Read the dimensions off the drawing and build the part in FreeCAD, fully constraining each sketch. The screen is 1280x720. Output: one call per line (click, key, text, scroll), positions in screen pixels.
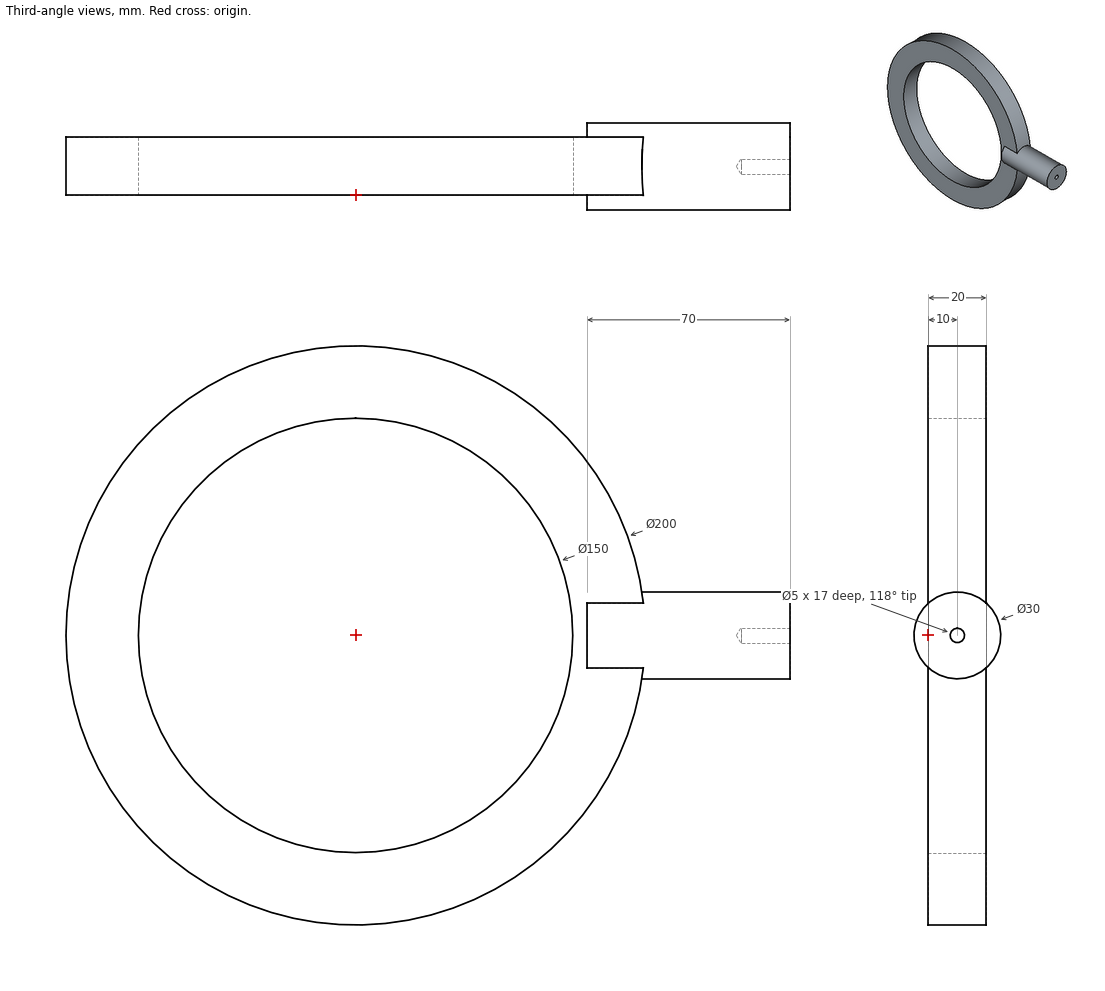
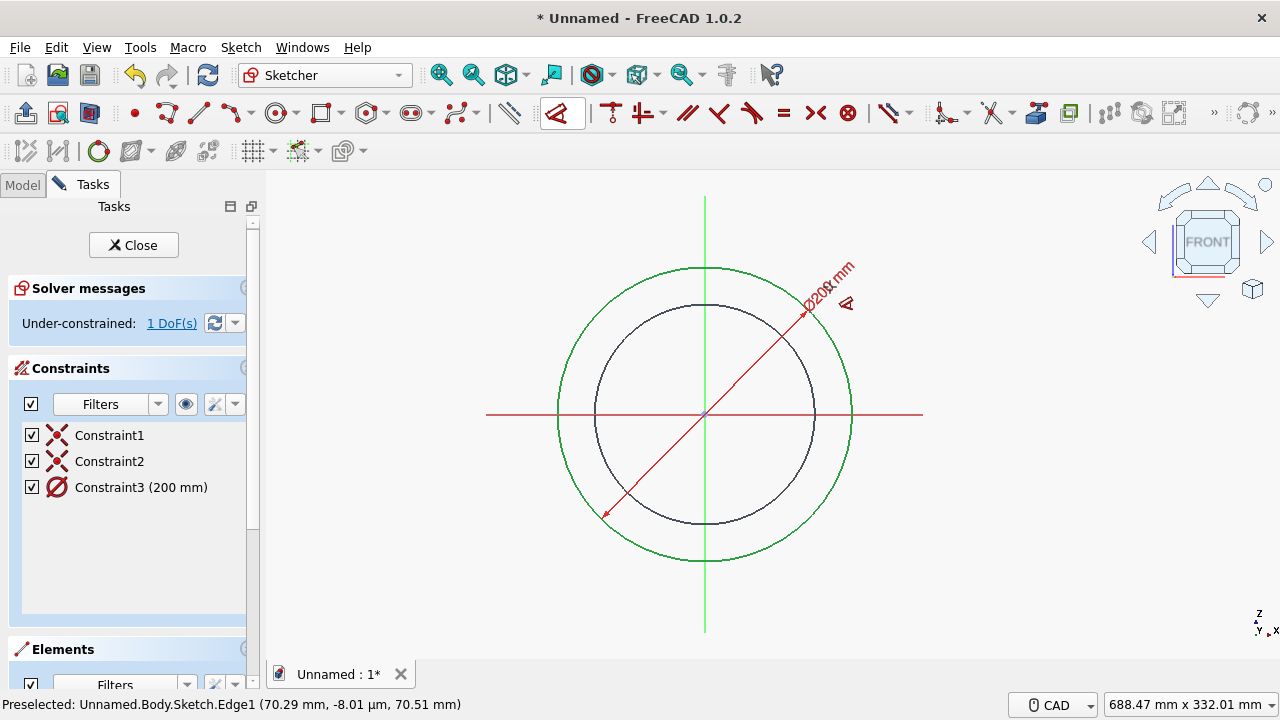
click(782, 336)
click(863, 367)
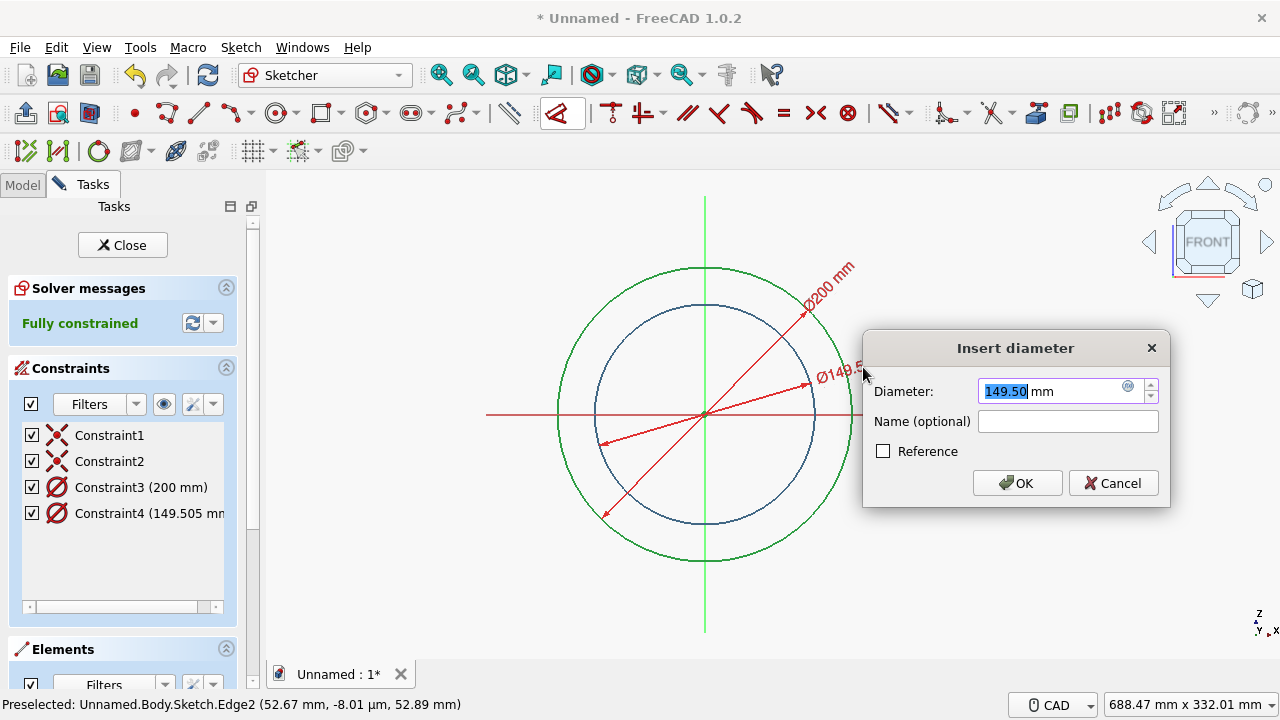
text(150)
key(Return)
key(Escape)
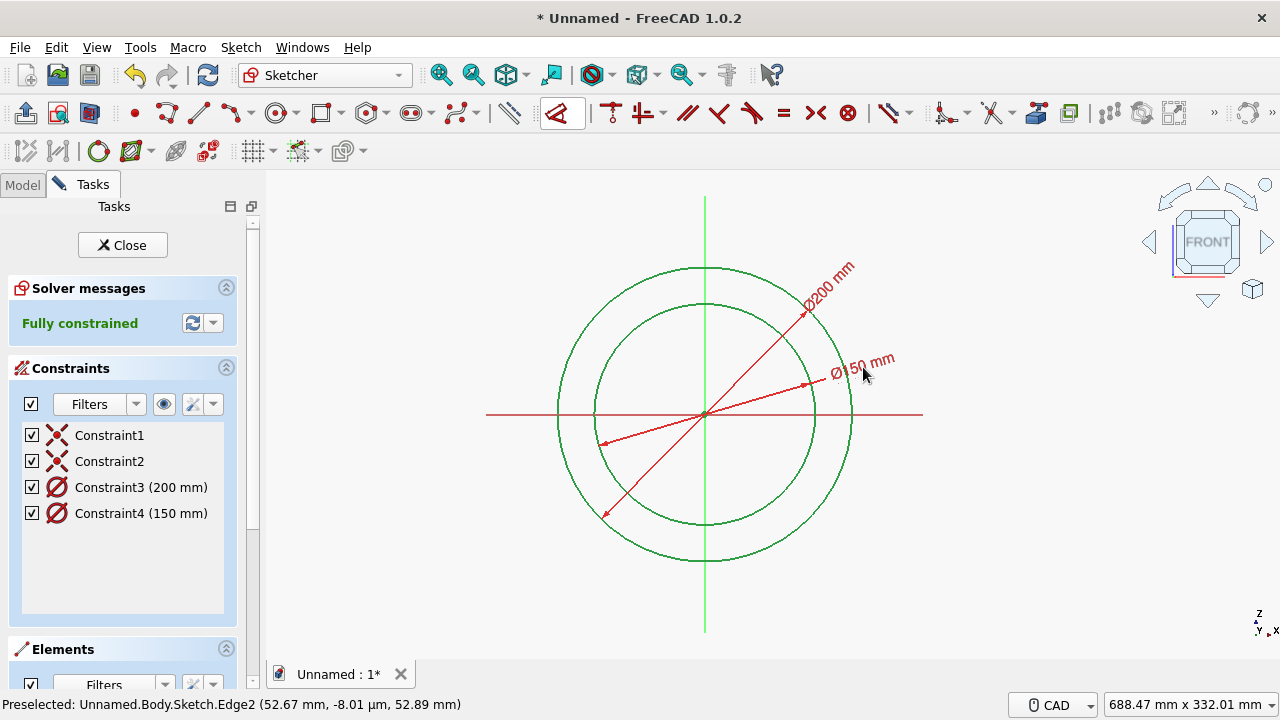
click(123, 245)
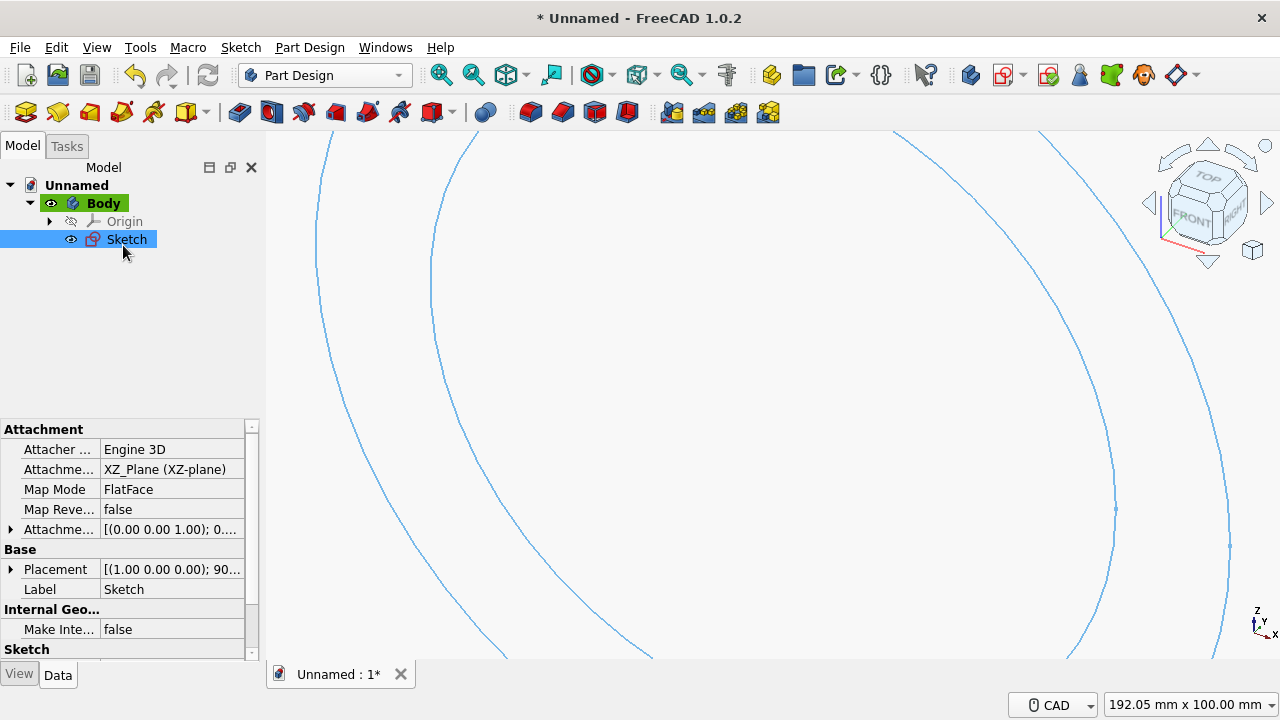
click(26, 112)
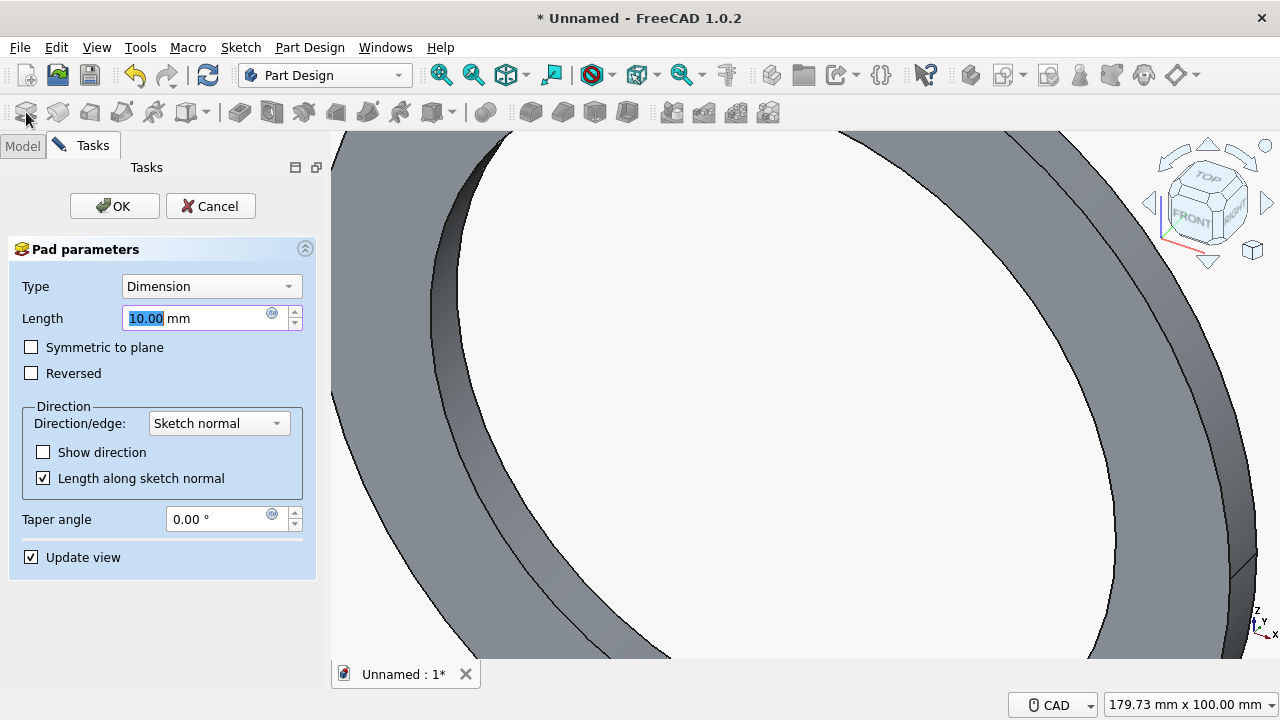
text(20)
key(Tab)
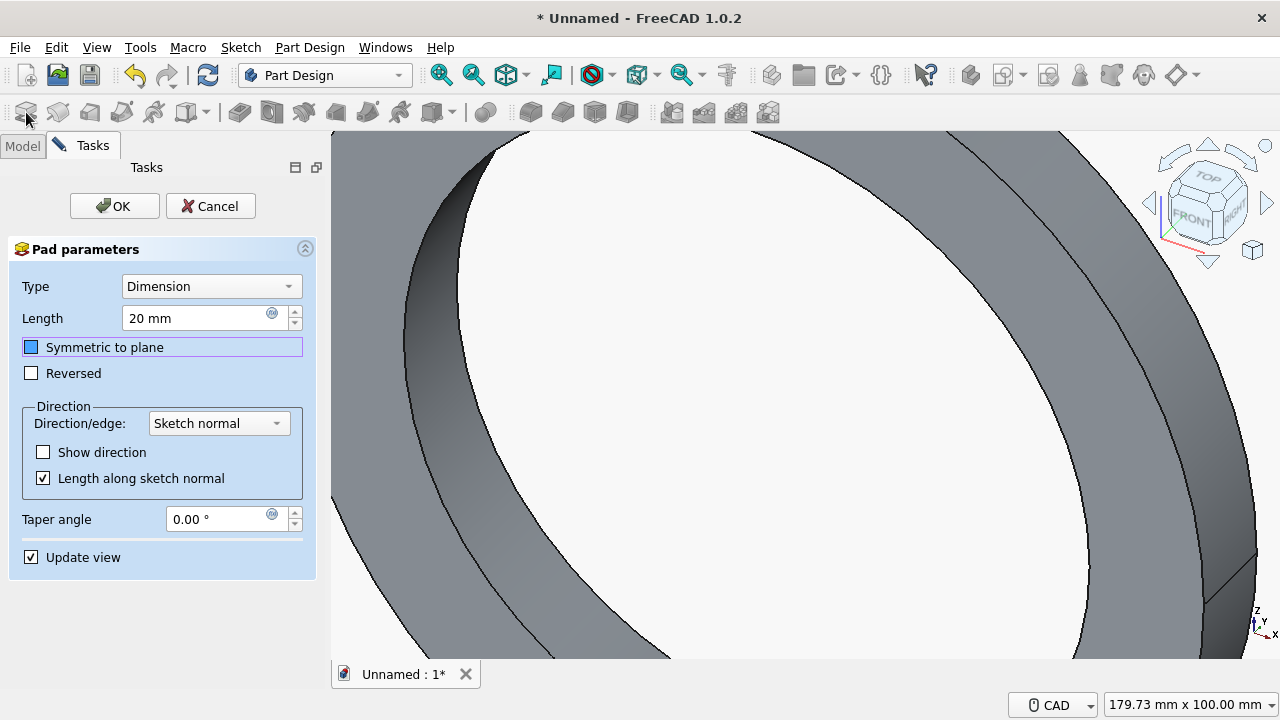
click(30, 373)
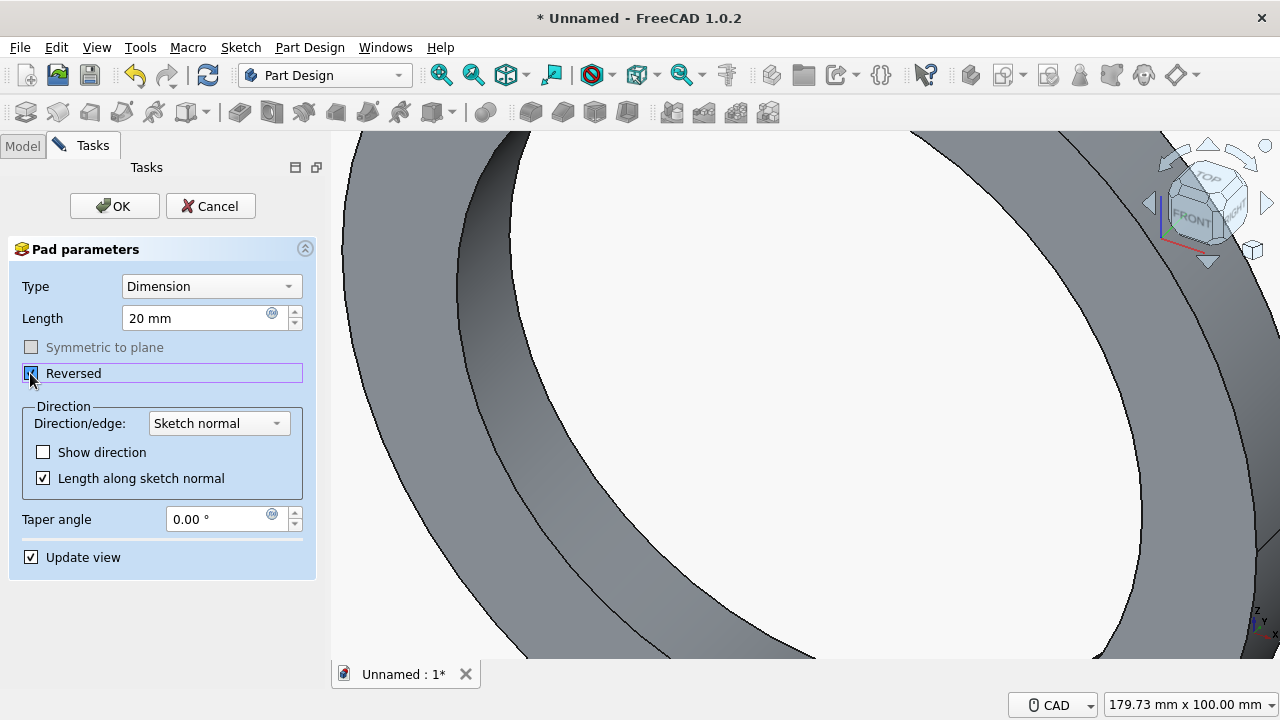
click(115, 206)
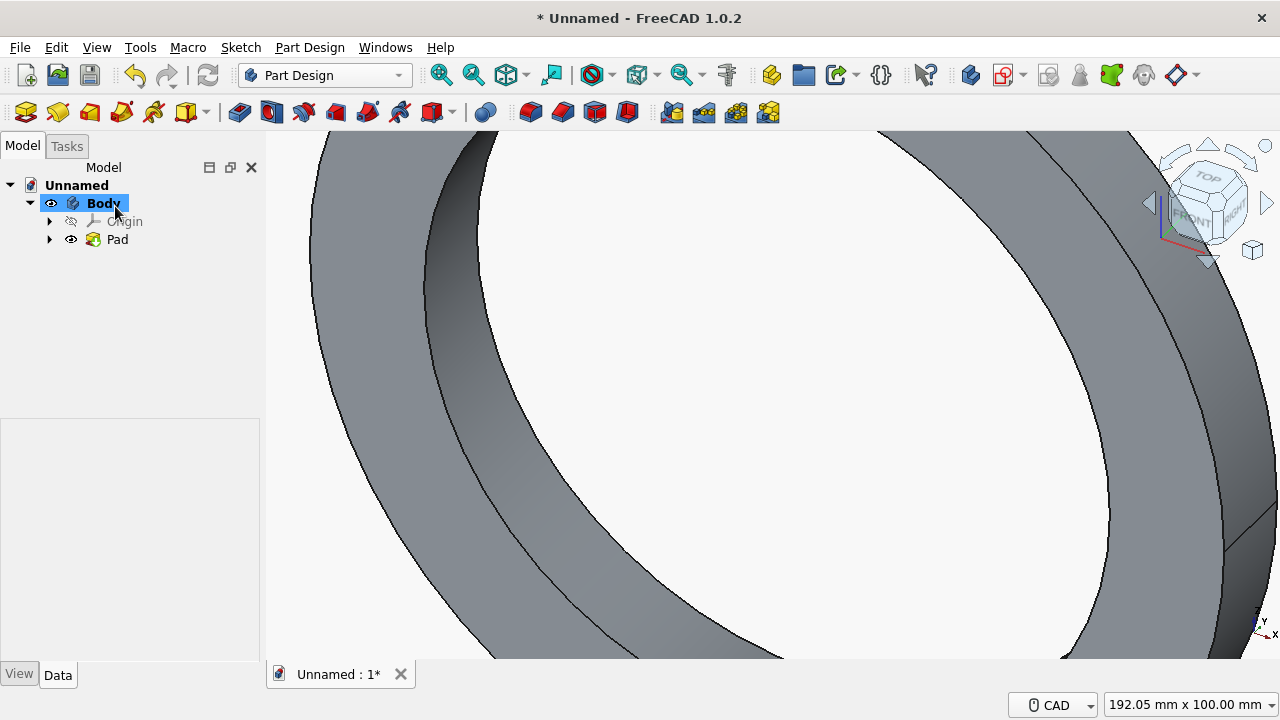
key(v)
key(f)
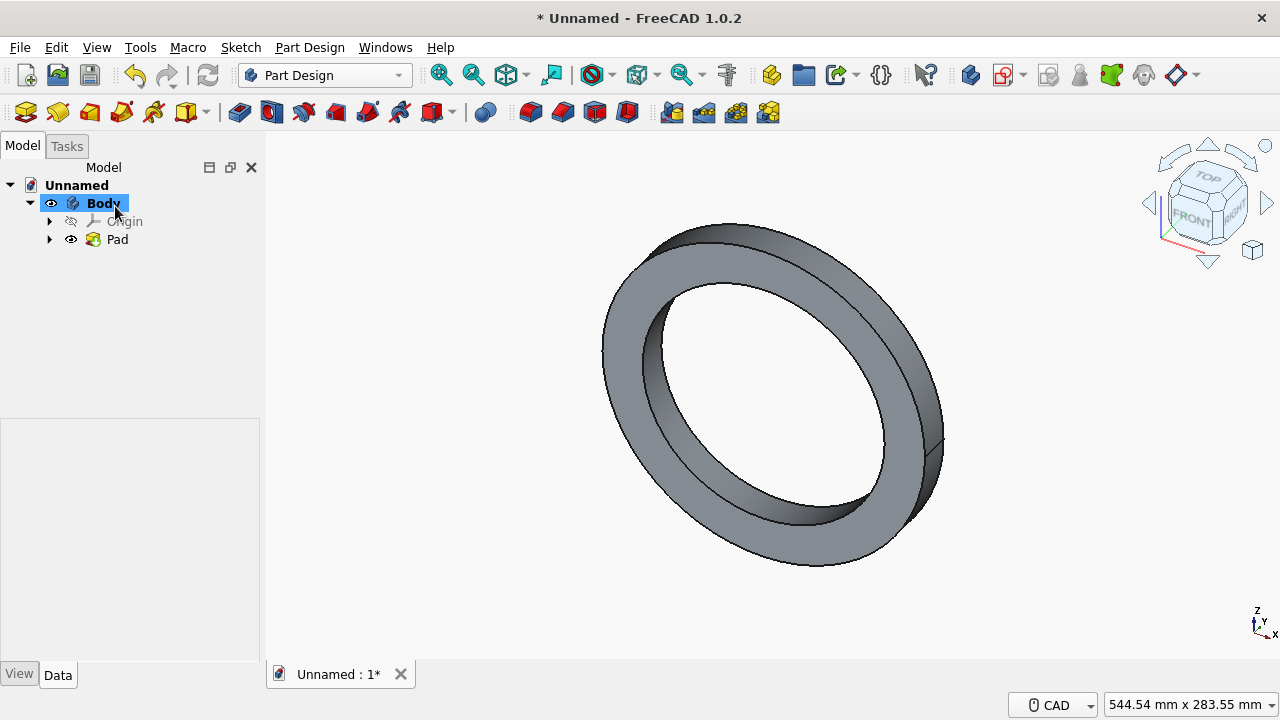
click(50, 221)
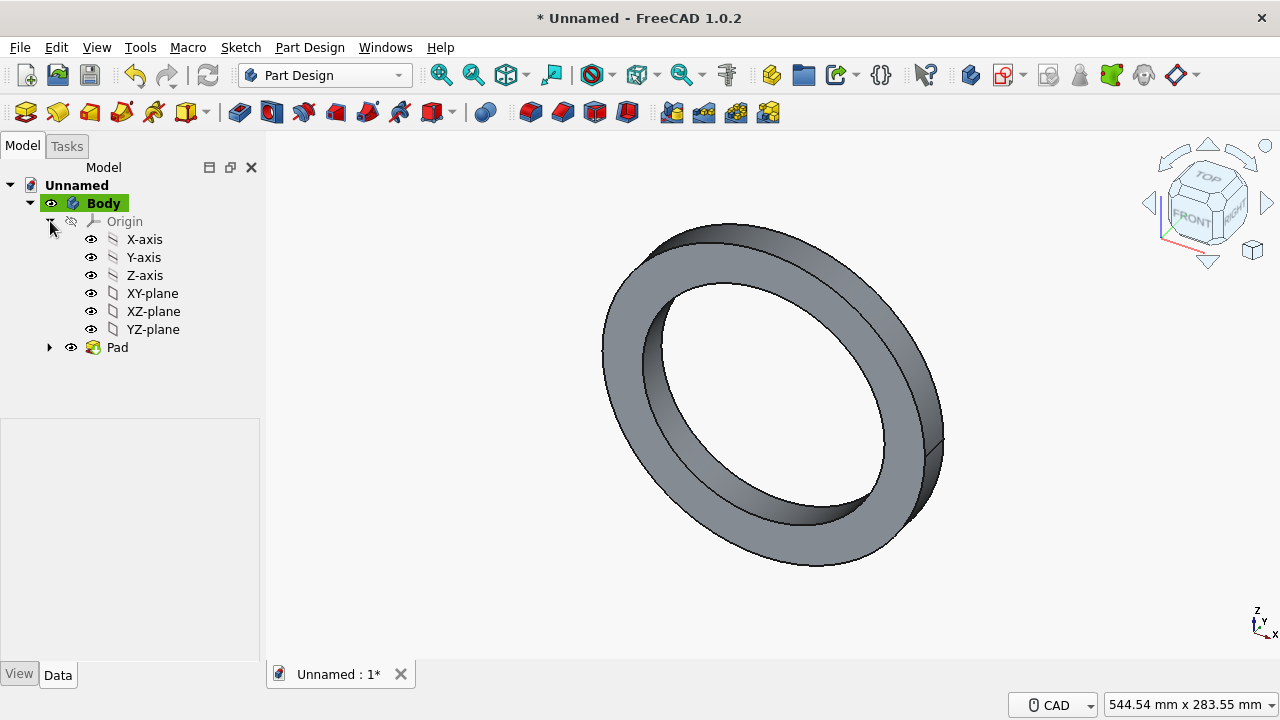
click(136, 329)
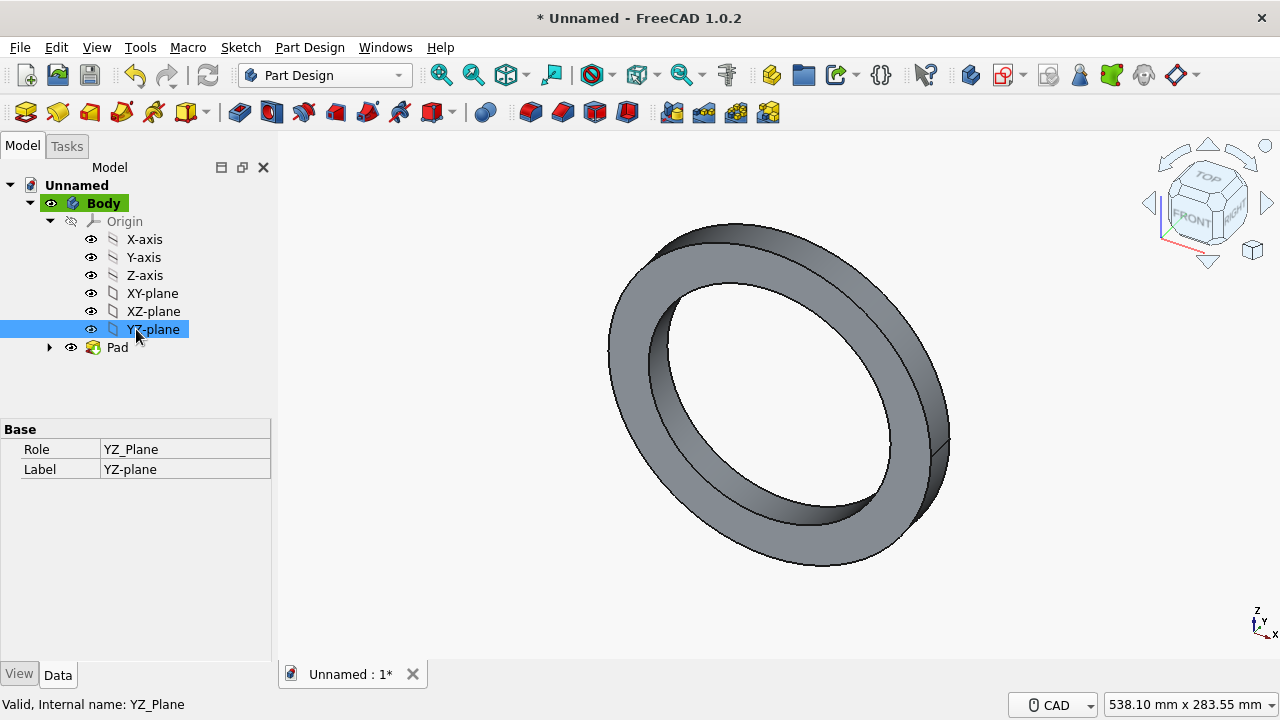
click(1176, 76)